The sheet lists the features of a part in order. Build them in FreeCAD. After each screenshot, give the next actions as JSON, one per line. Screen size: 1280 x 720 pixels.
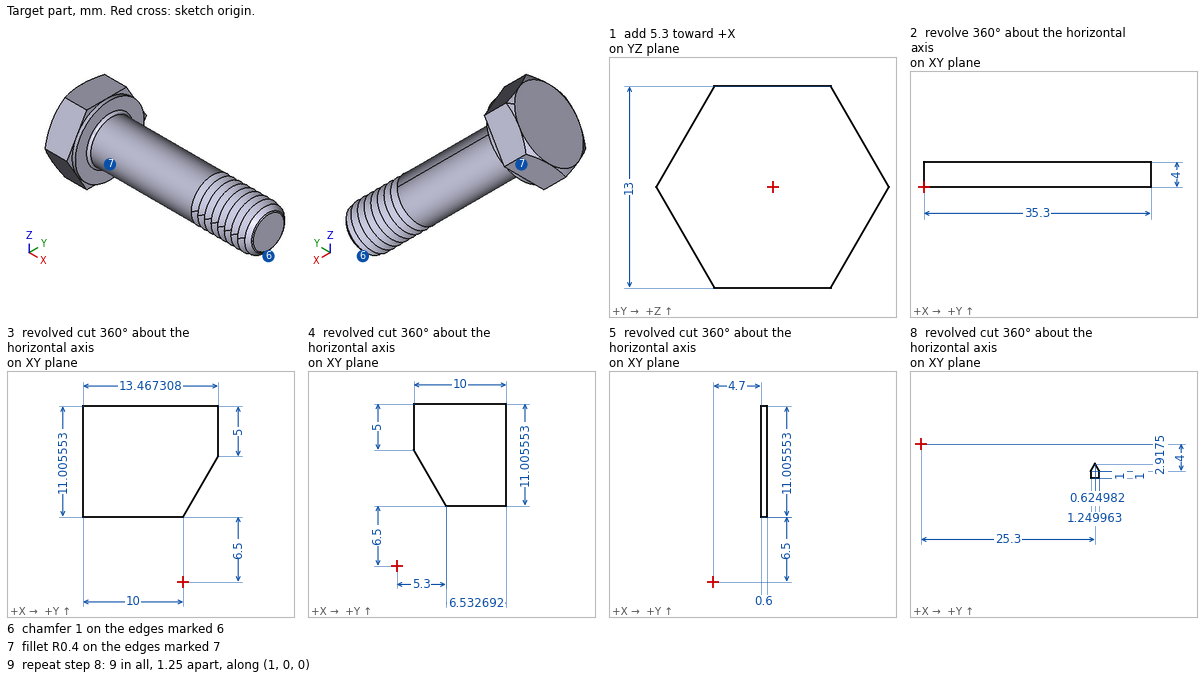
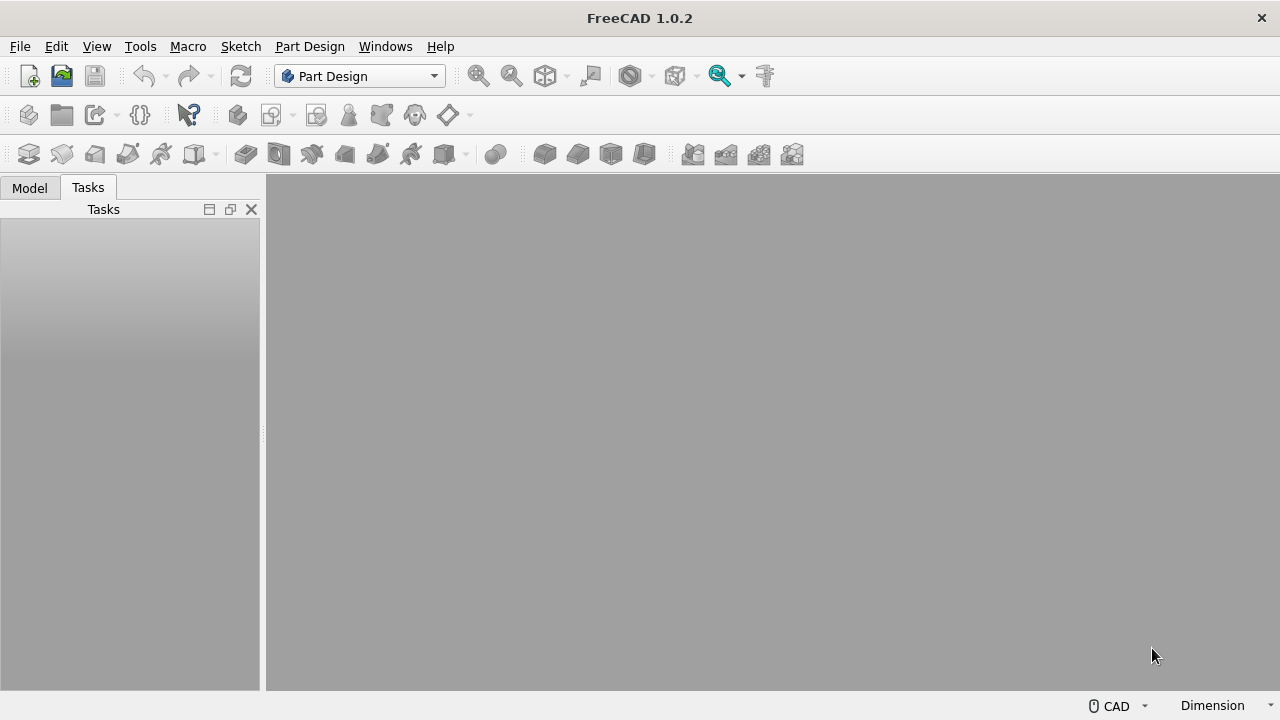
{"action": "left_click", "coordinate": [29, 76]}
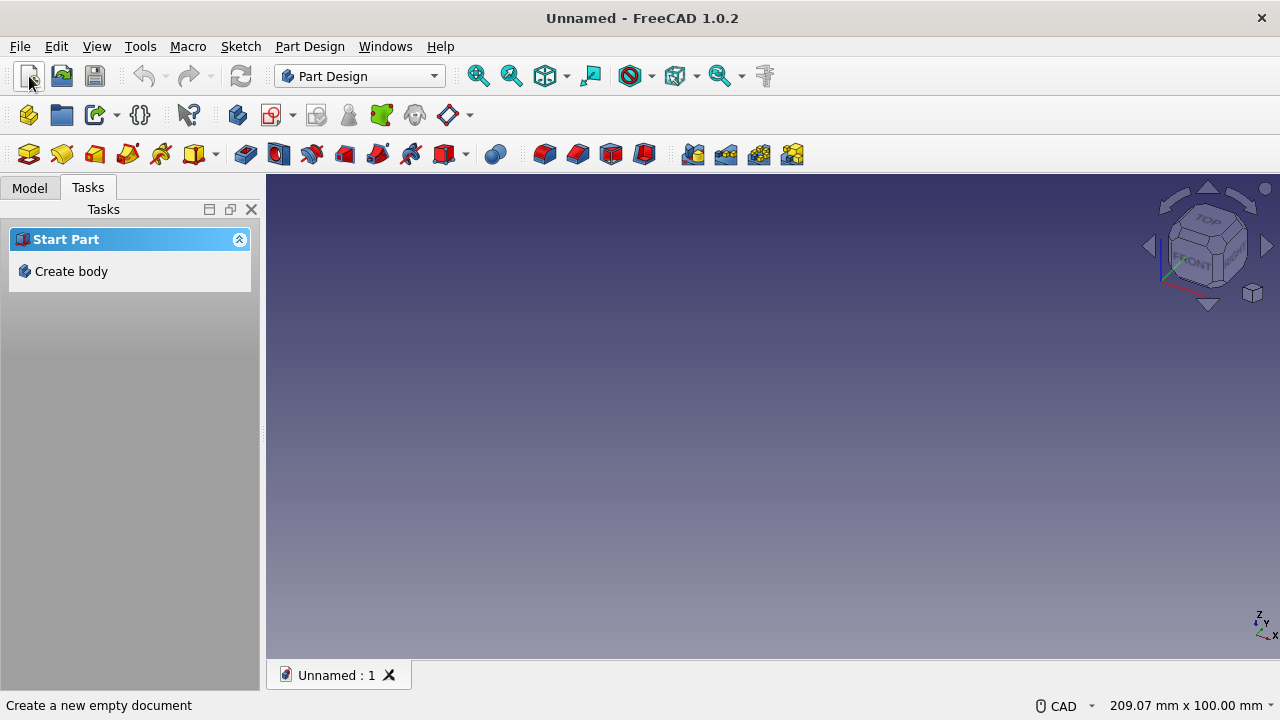
{"action": "left_click", "coordinate": [270, 116]}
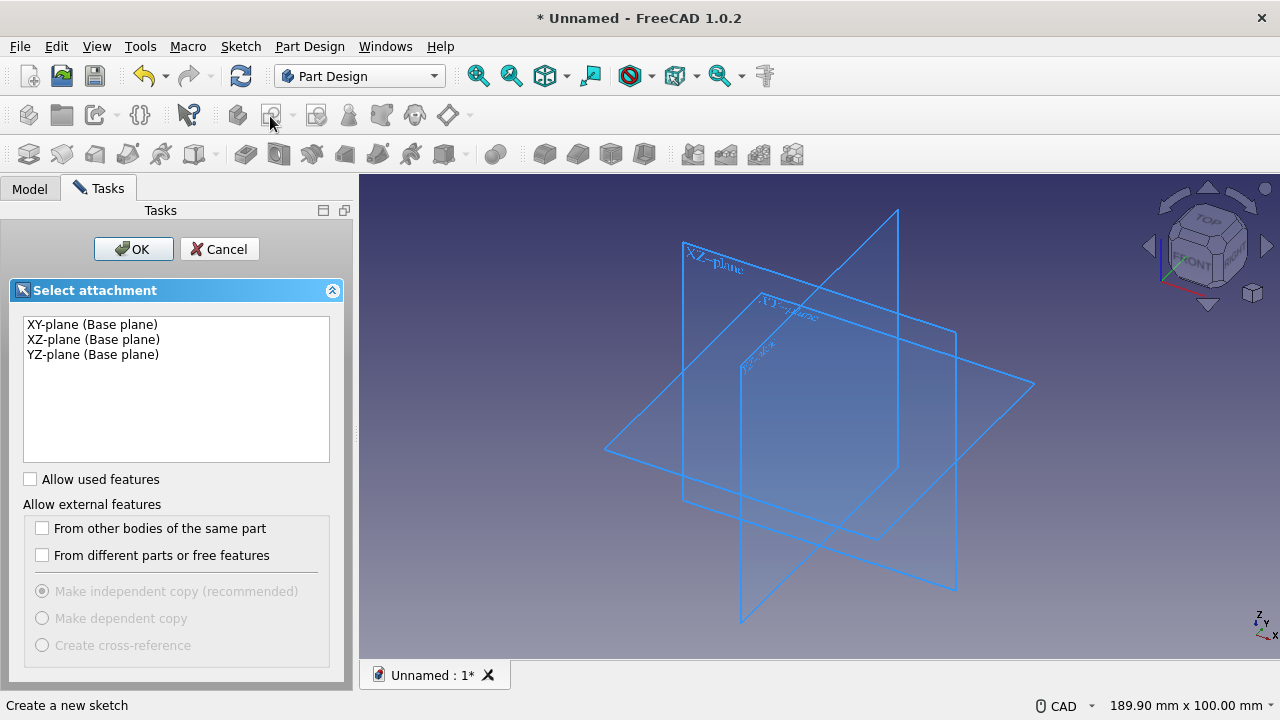
{"action": "left_click", "coordinate": [84, 354]}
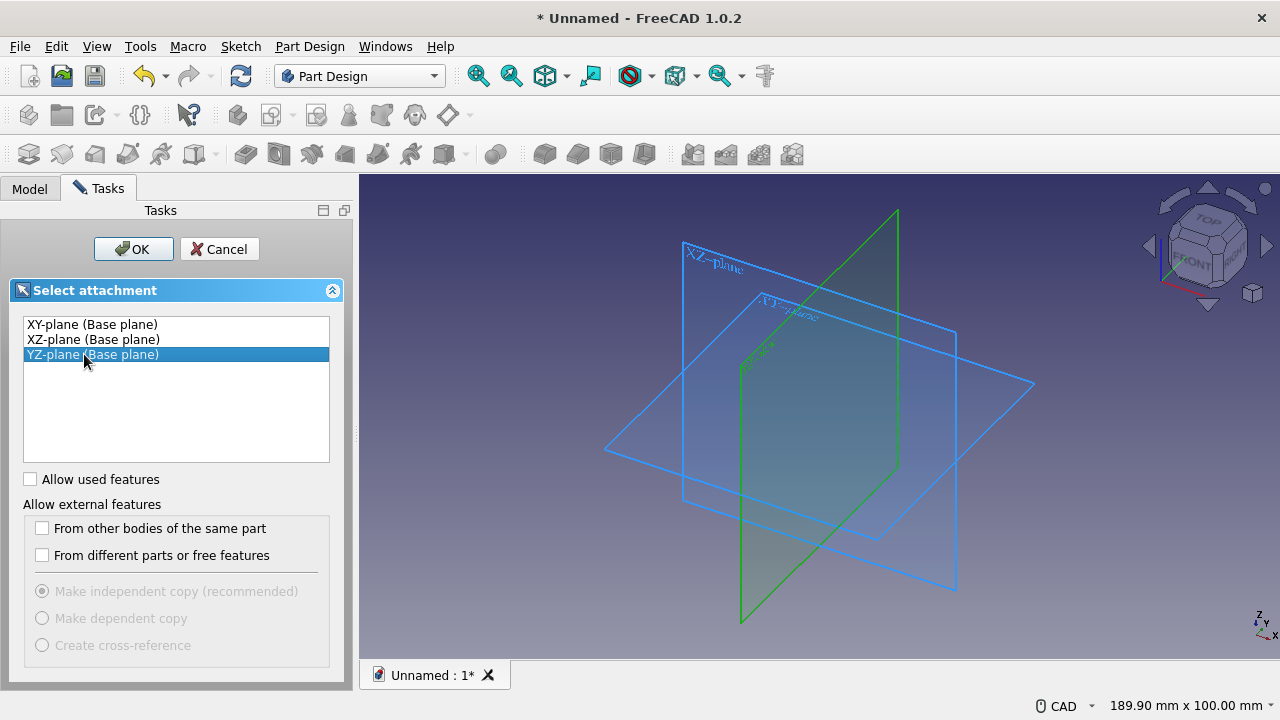
{"action": "left_click", "coordinate": [134, 249]}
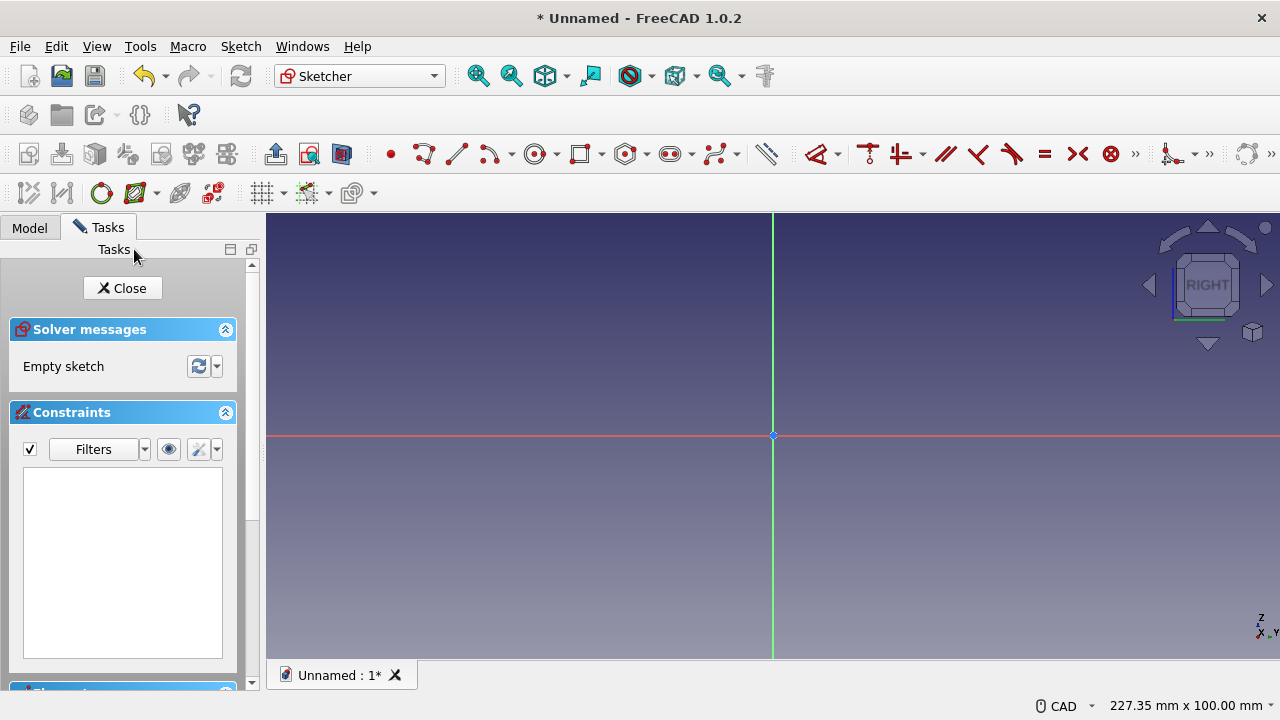
{"action": "scroll", "coordinate": [790, 436], "scroll_direction": "up", "scroll_amount": 8}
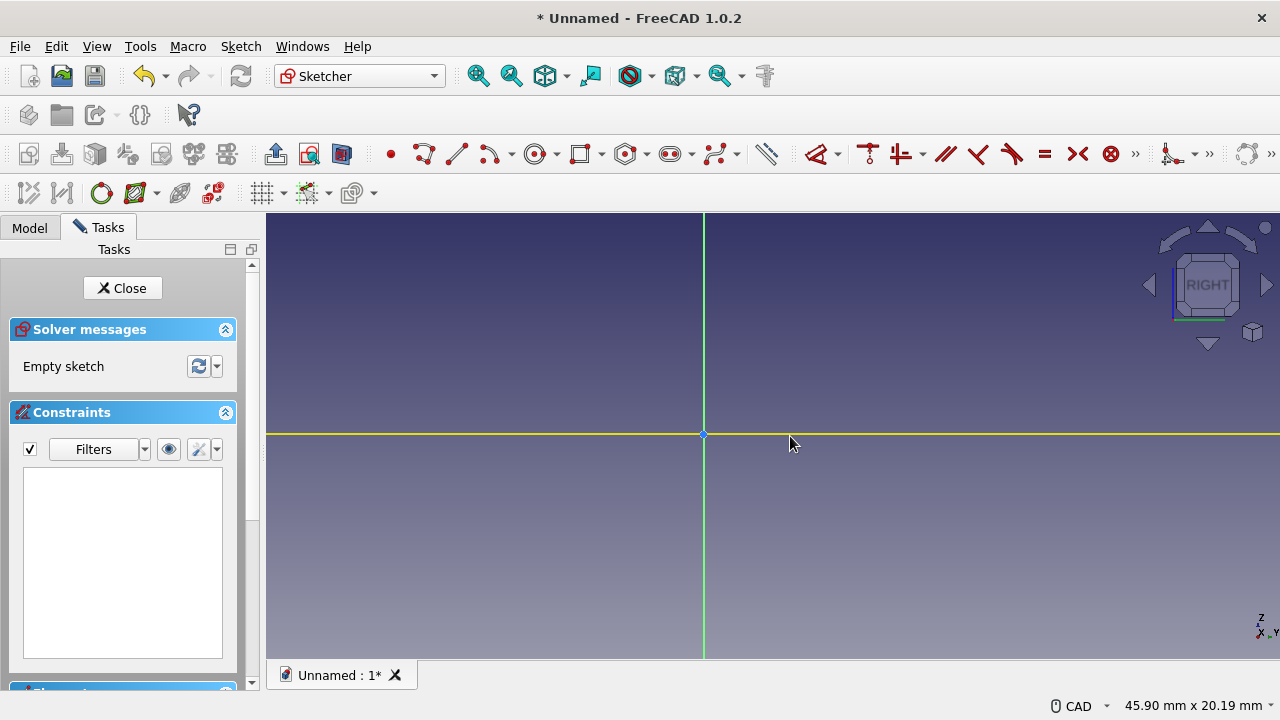
{"action": "left_click", "coordinate": [624, 154]}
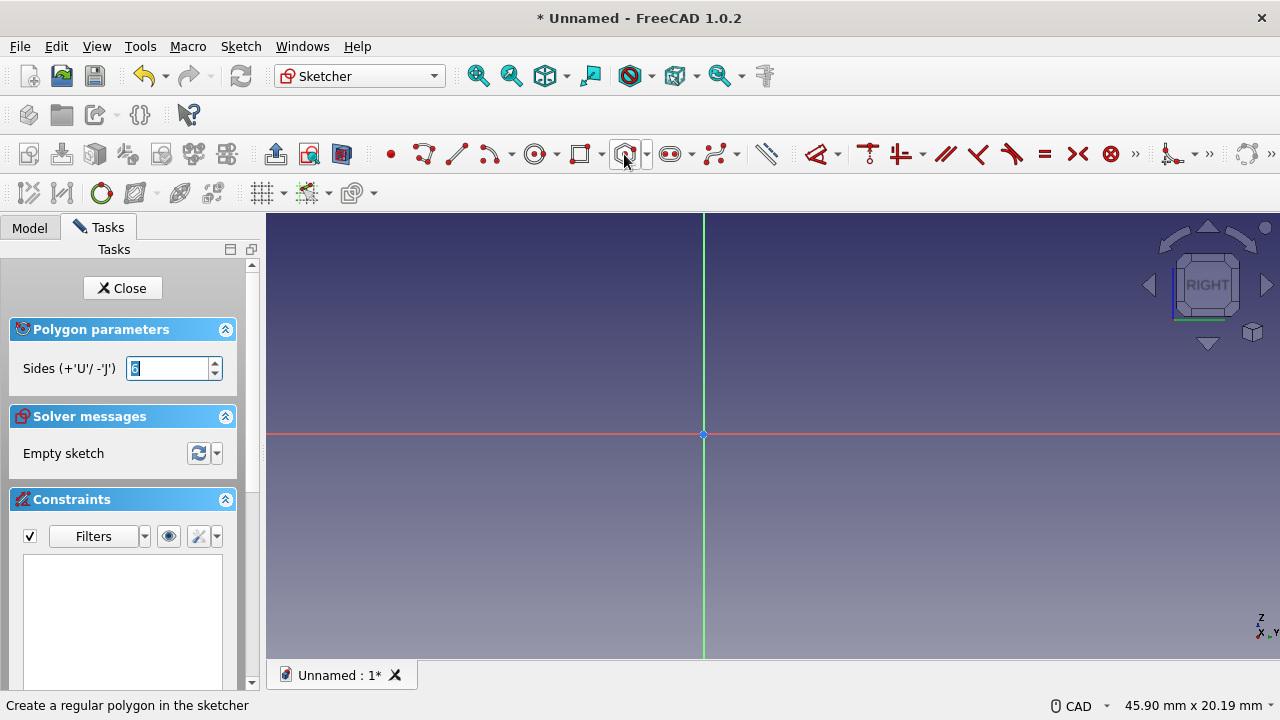
{"action": "left_click", "coordinate": [704, 434]}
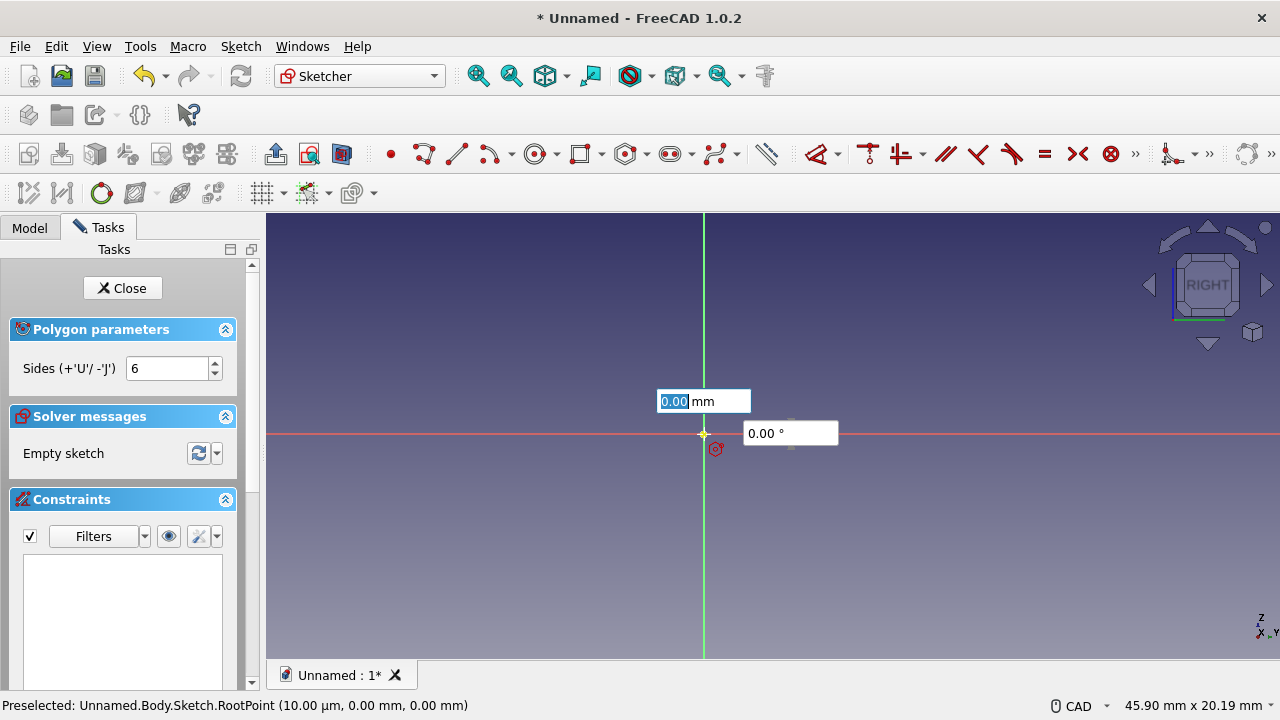
{"action": "left_click", "coordinate": [870, 434]}
{"action": "right_click", "coordinate": [870, 434]}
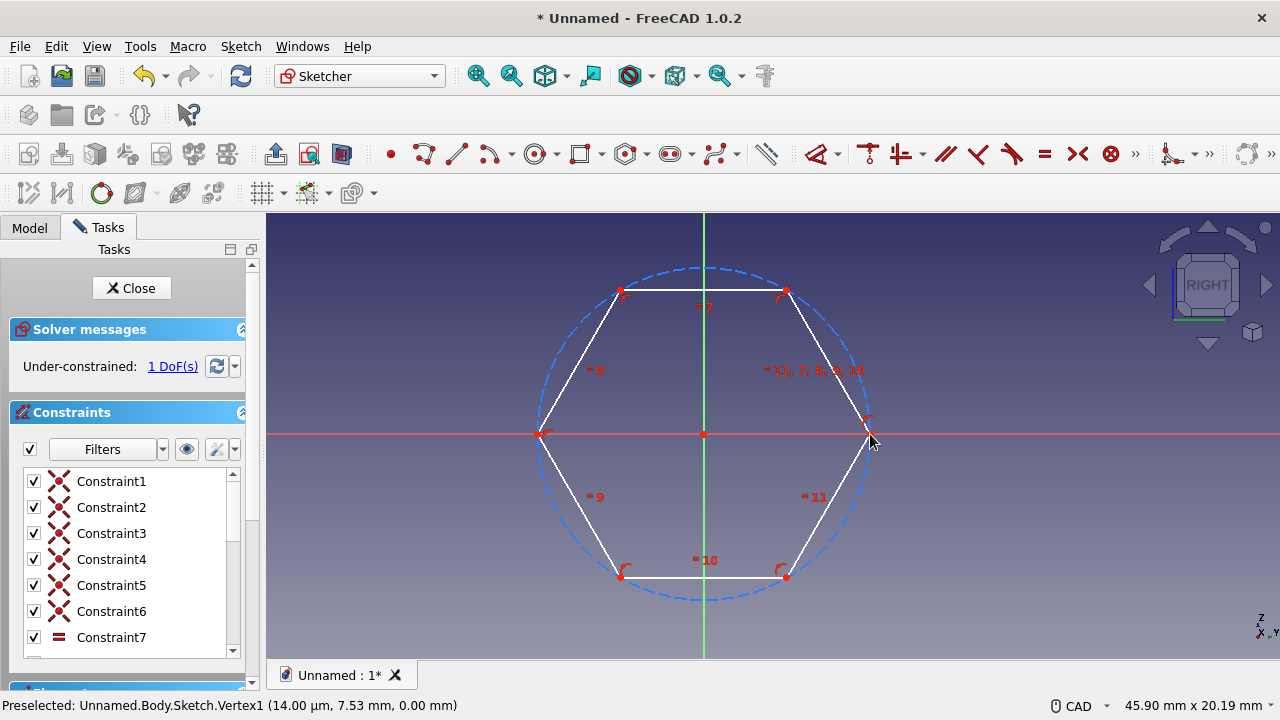
{"action": "left_click", "coordinate": [816, 154]}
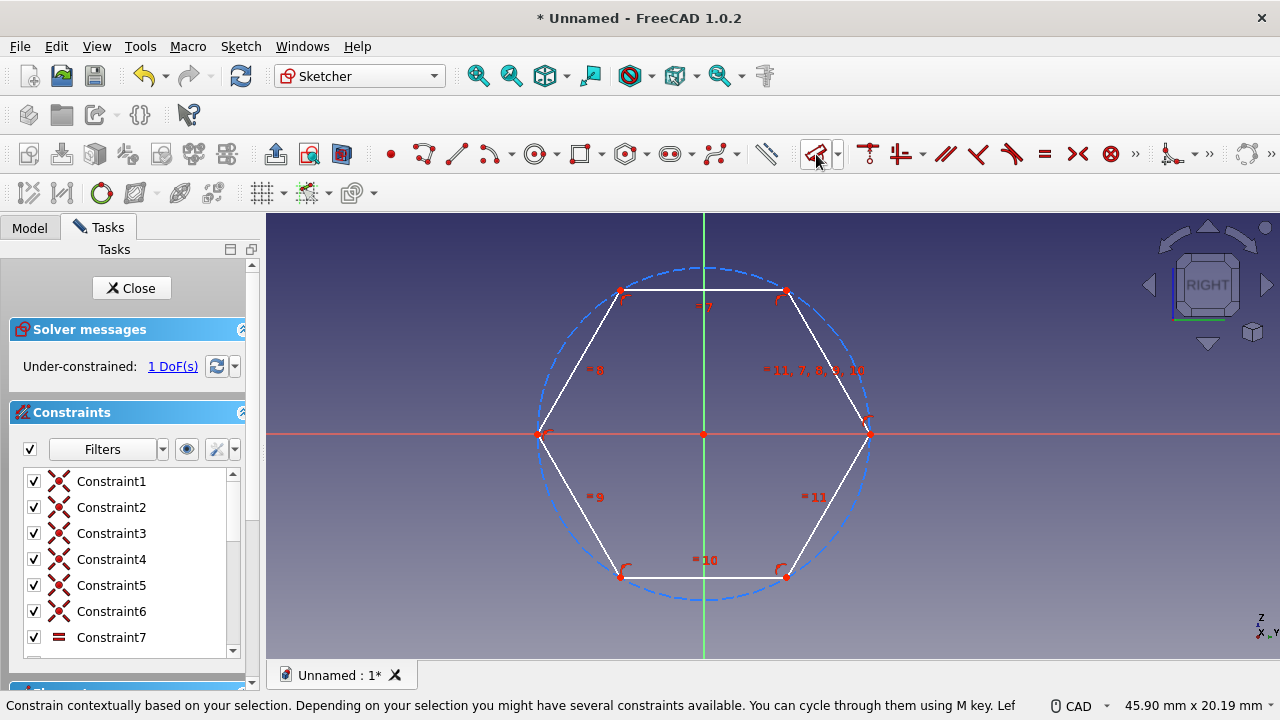
{"action": "left_click", "coordinate": [621, 578]}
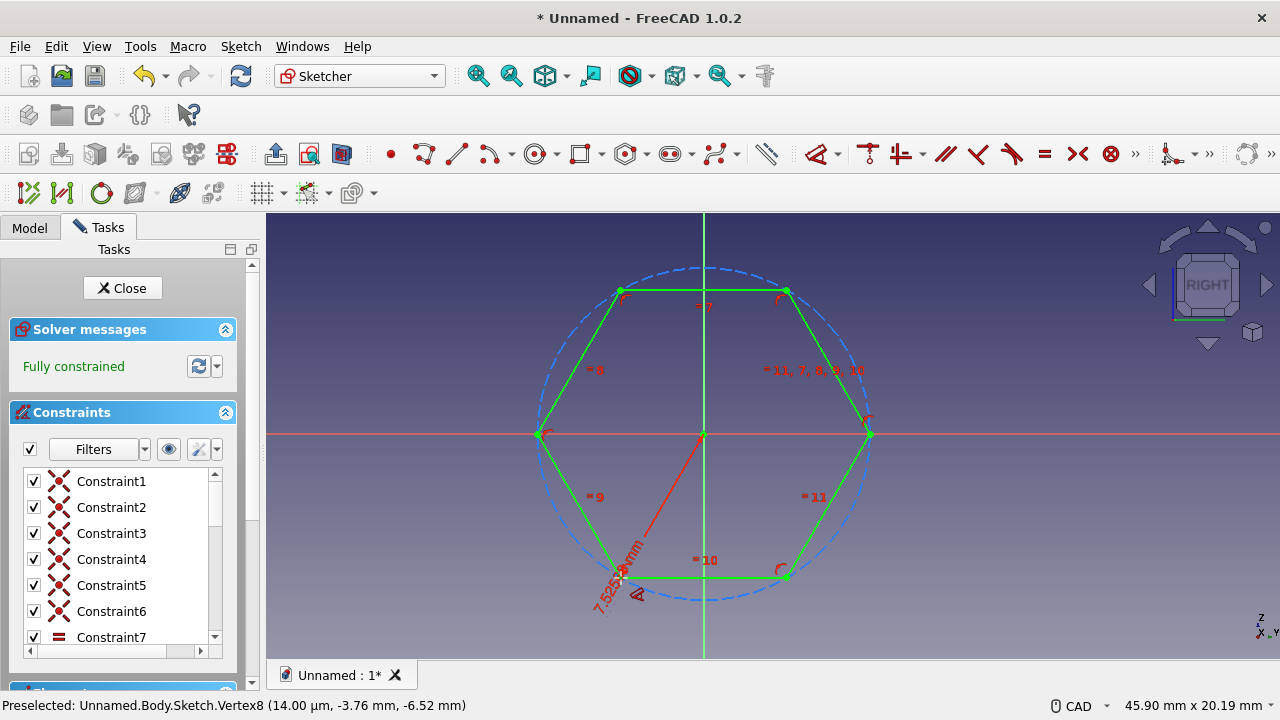
{"action": "left_click", "coordinate": [787, 290]}
{"action": "left_click", "coordinate": [869, 333]}